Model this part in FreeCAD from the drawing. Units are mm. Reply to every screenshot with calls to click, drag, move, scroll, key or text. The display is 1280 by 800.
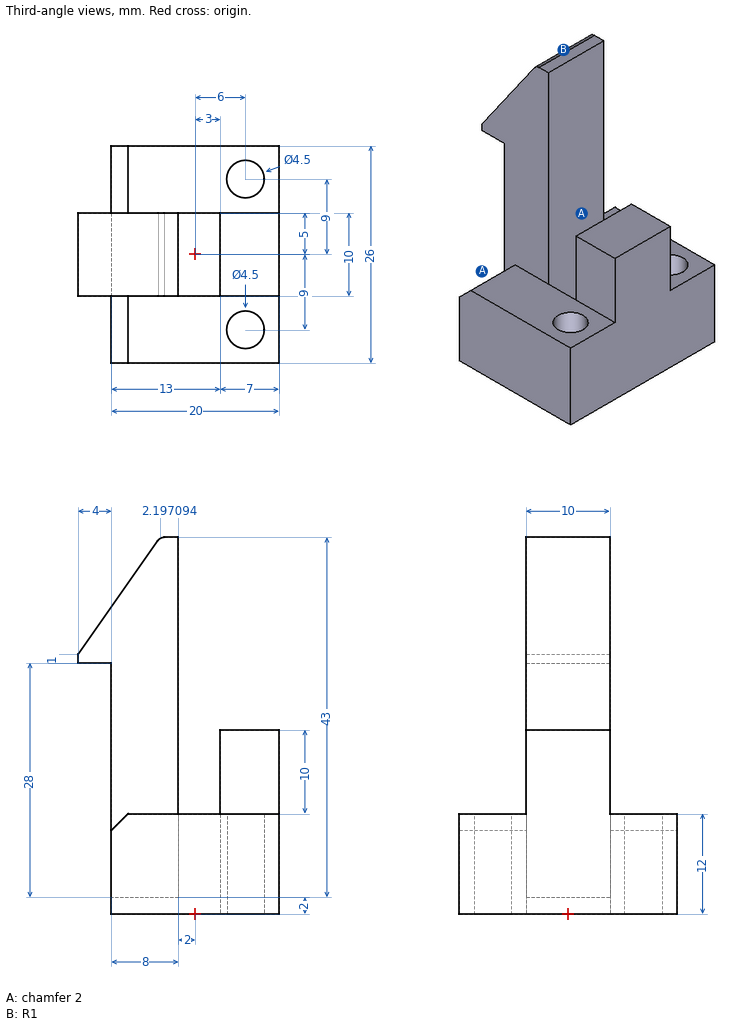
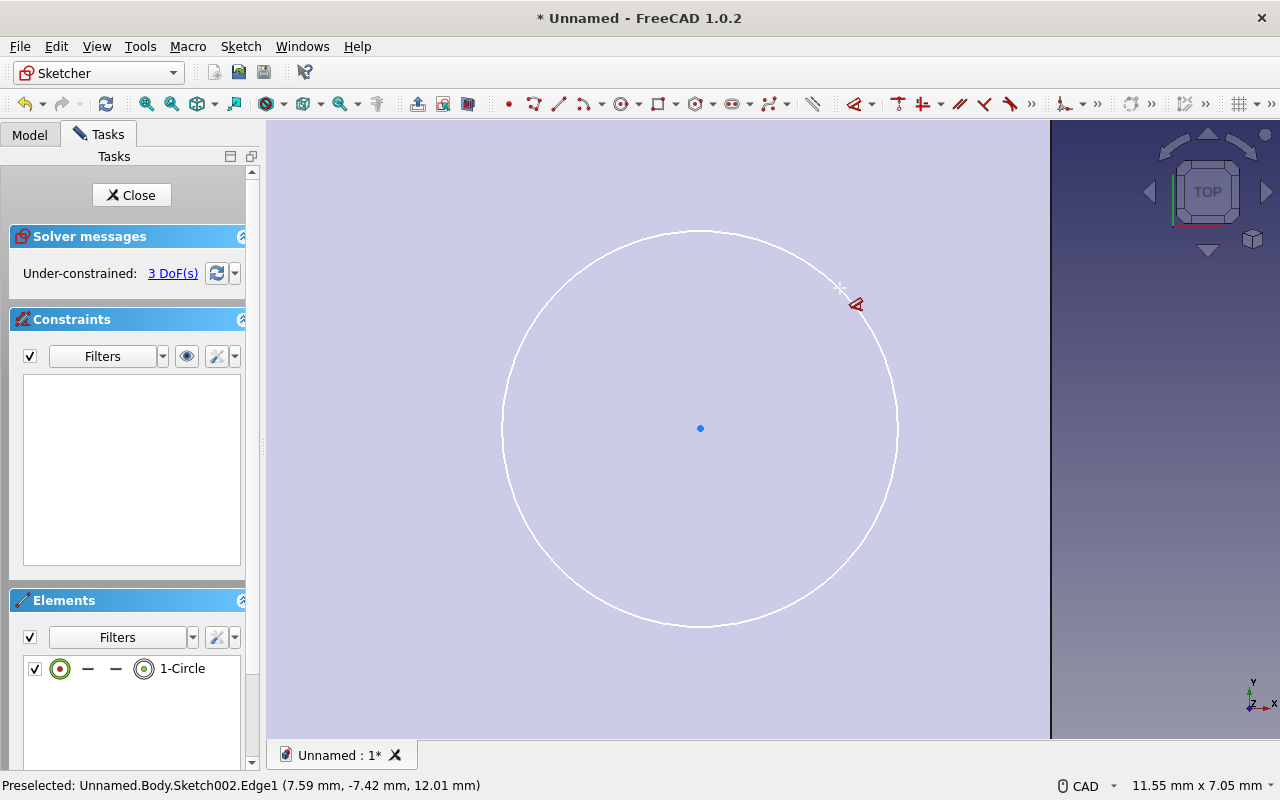
click(840, 289)
click(863, 266)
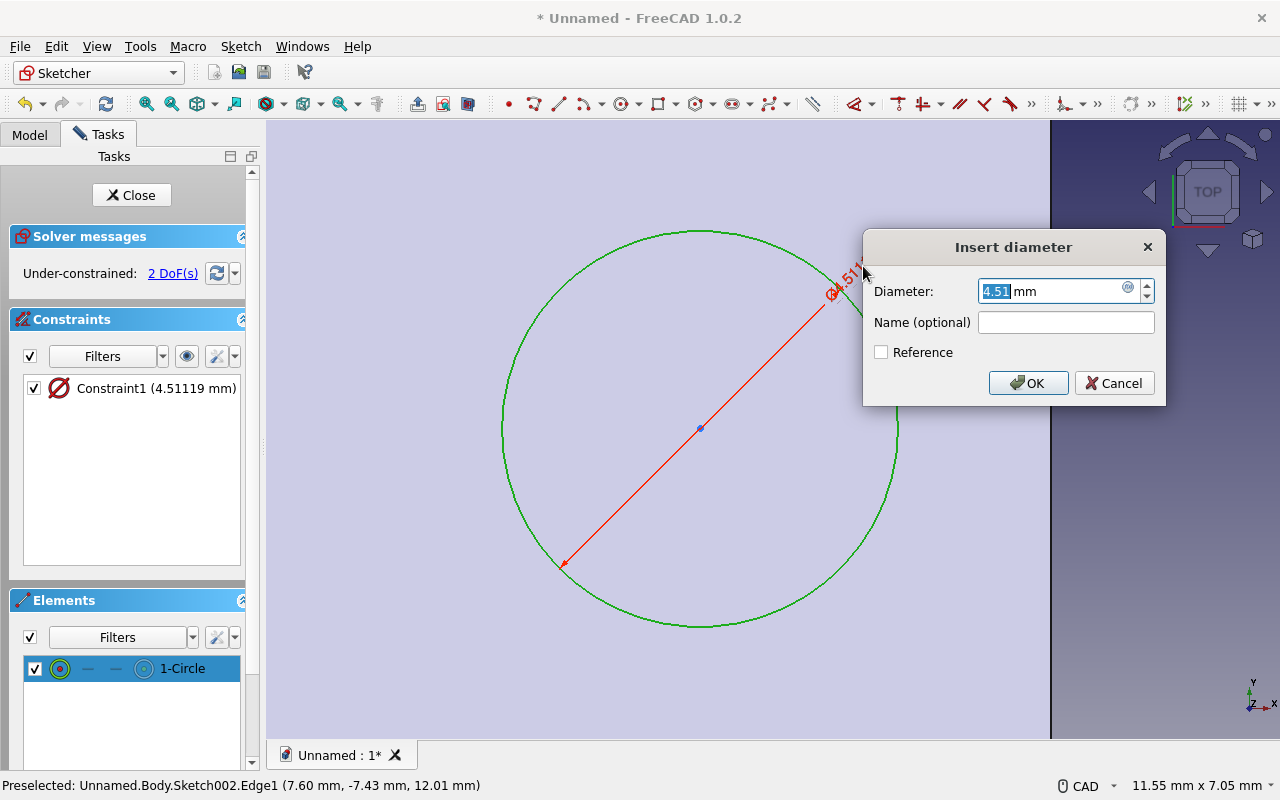
text(4.5)
key(Return)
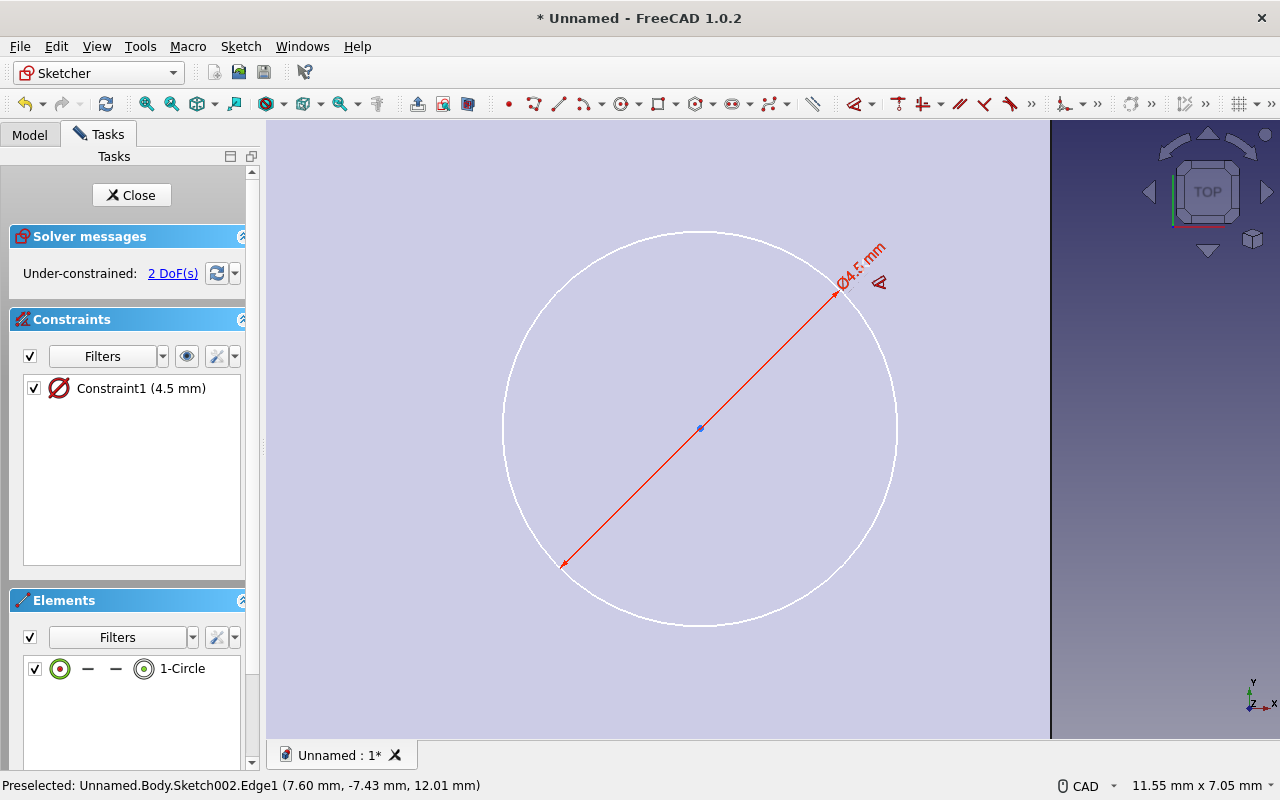
click(700, 429)
click(404, 463)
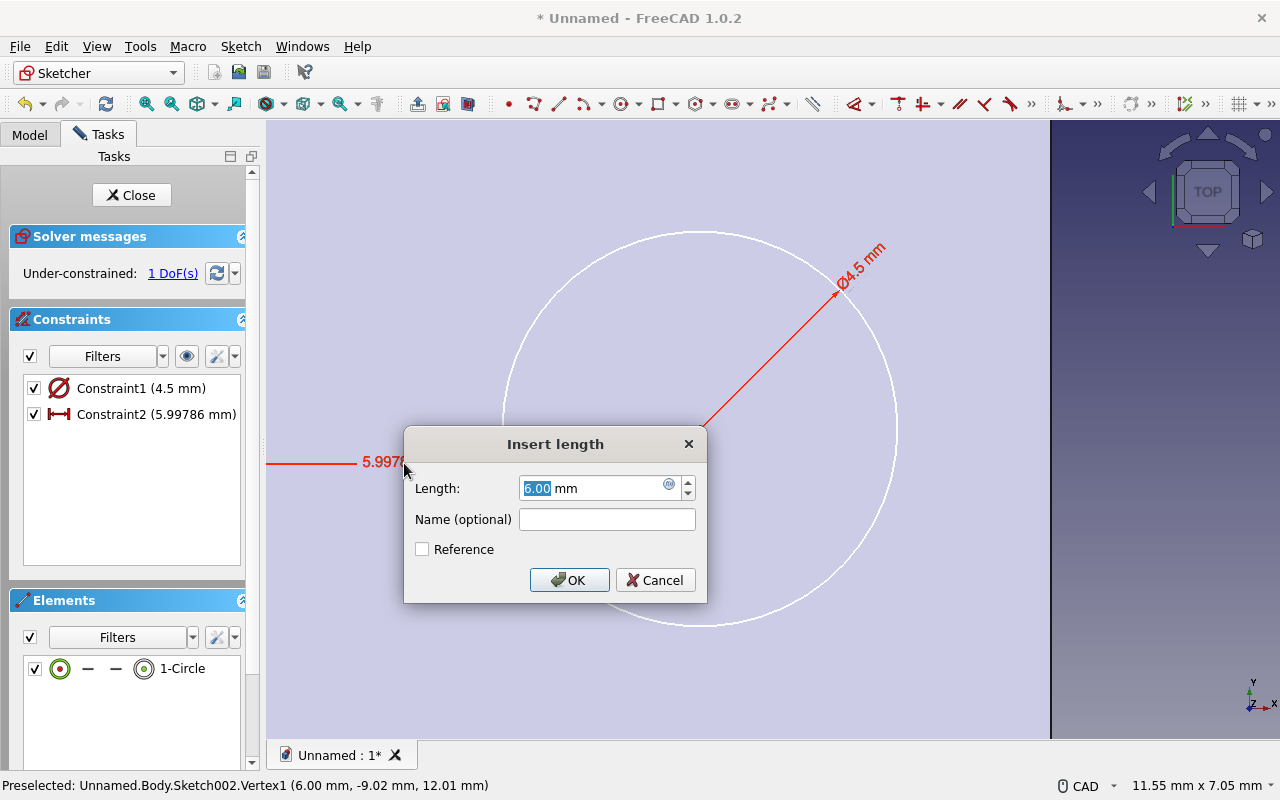
text(6)
key(Return)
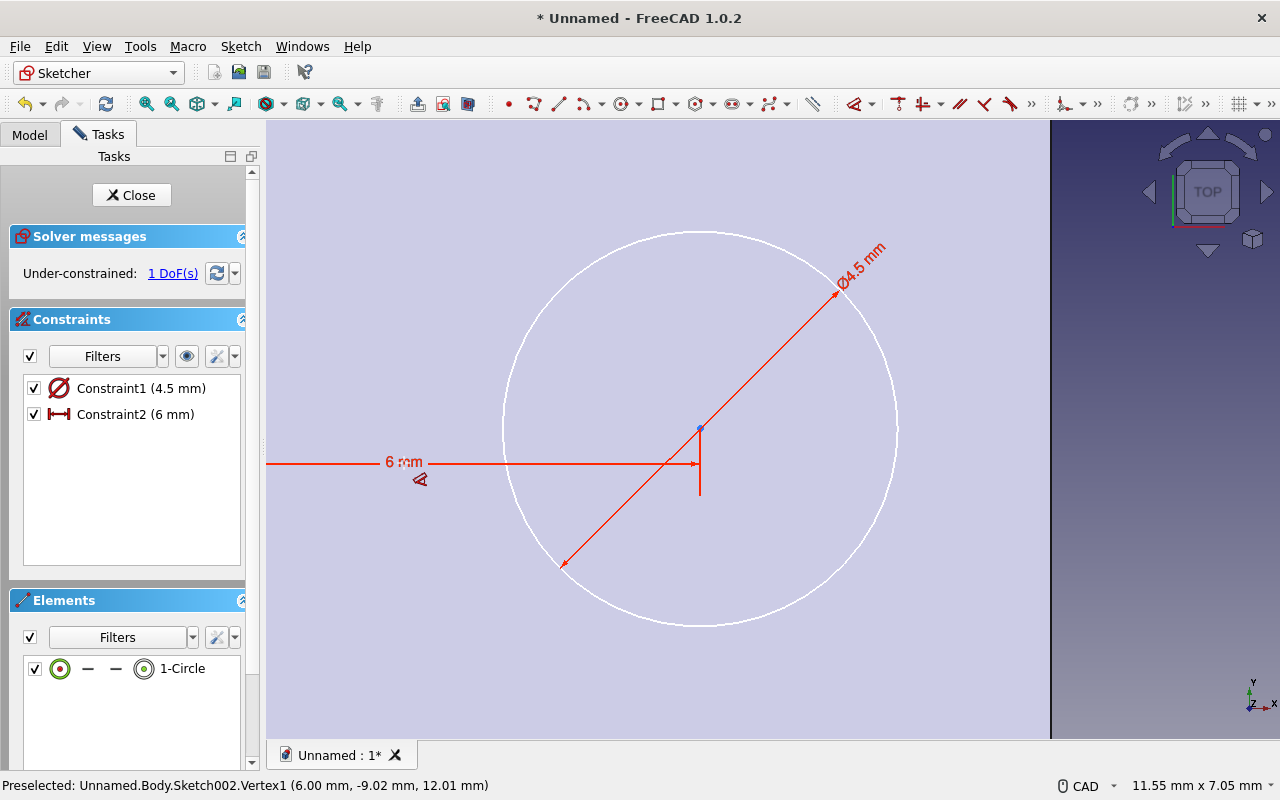
click(700, 429)
click(734, 288)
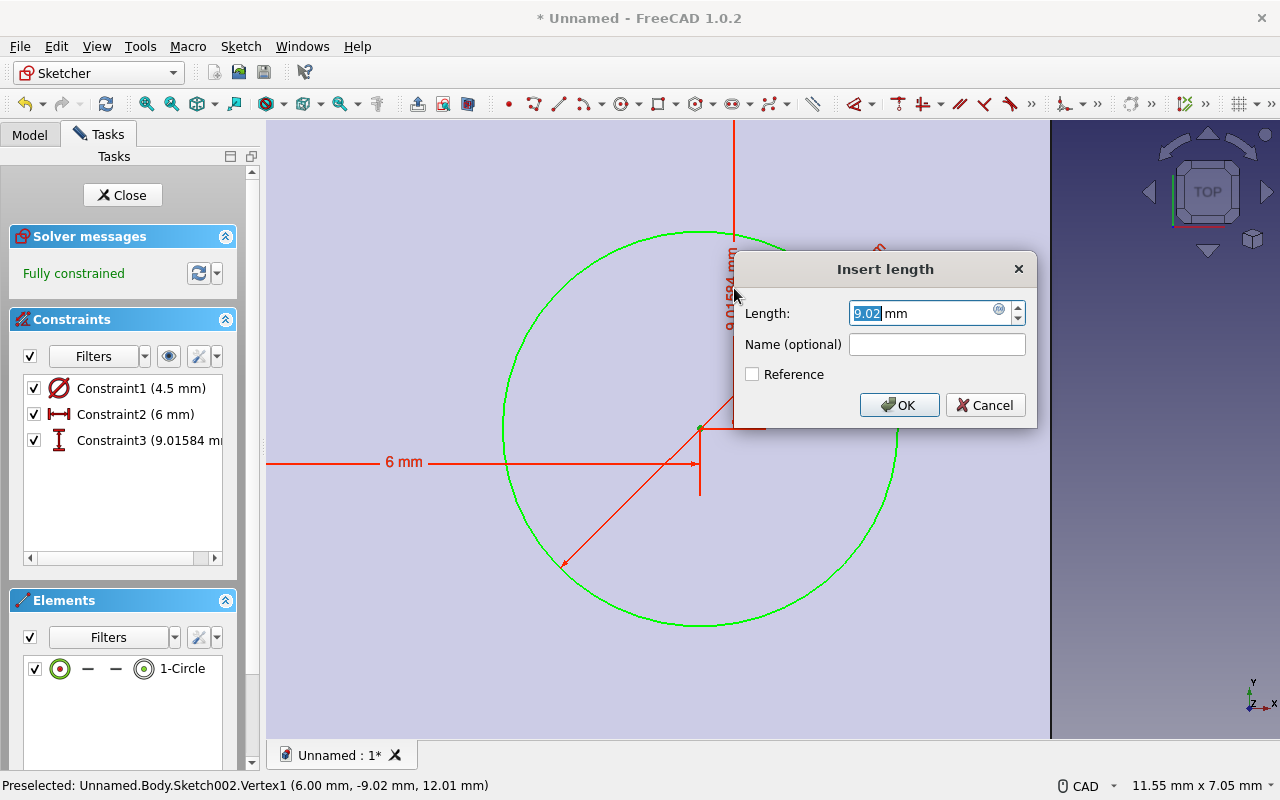
text(9)
key(Return)
key(Escape)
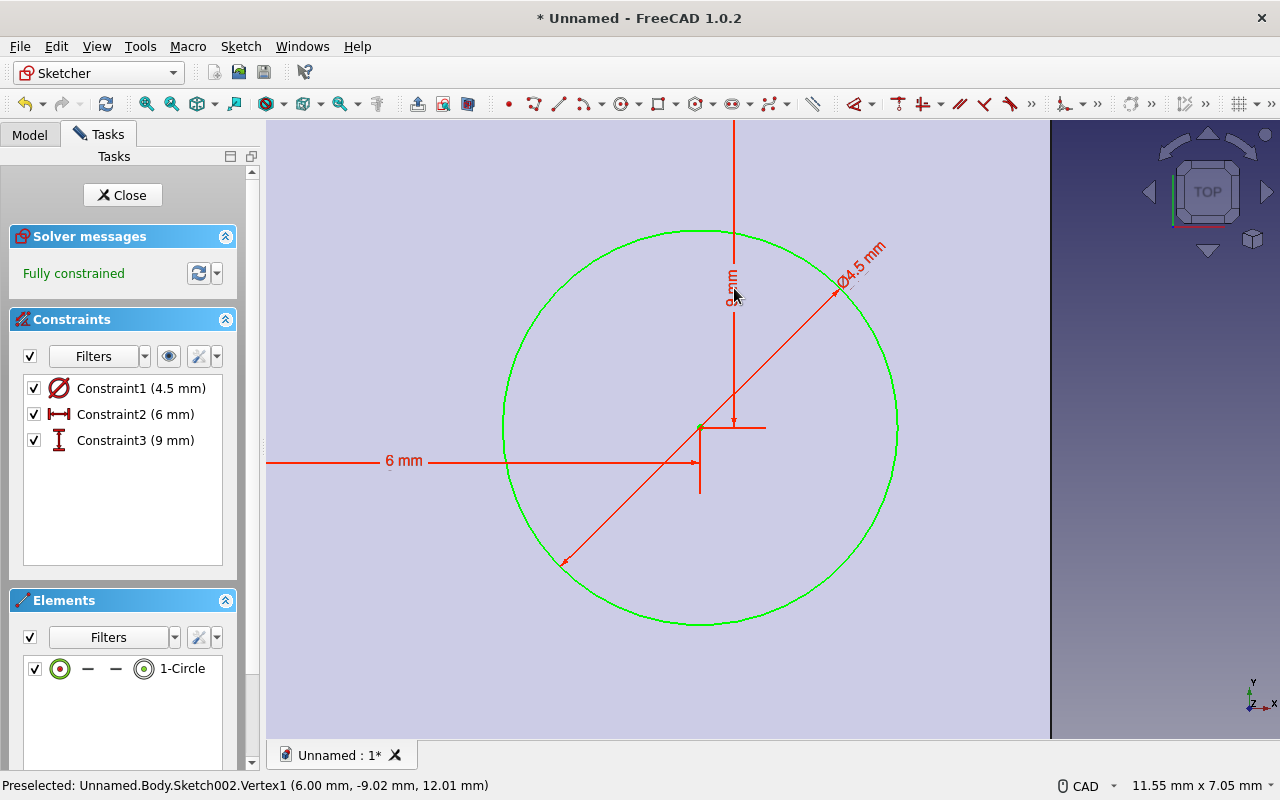
click(123, 195)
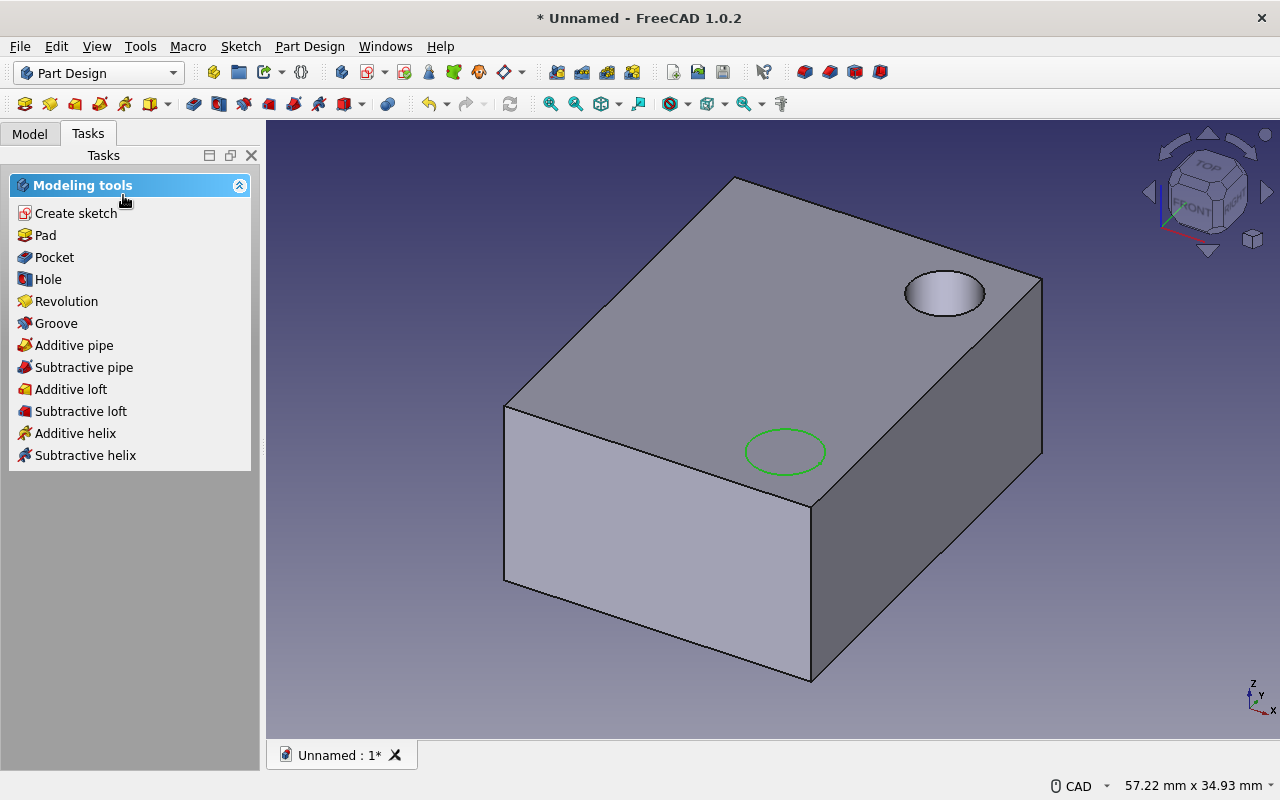
click(194, 104)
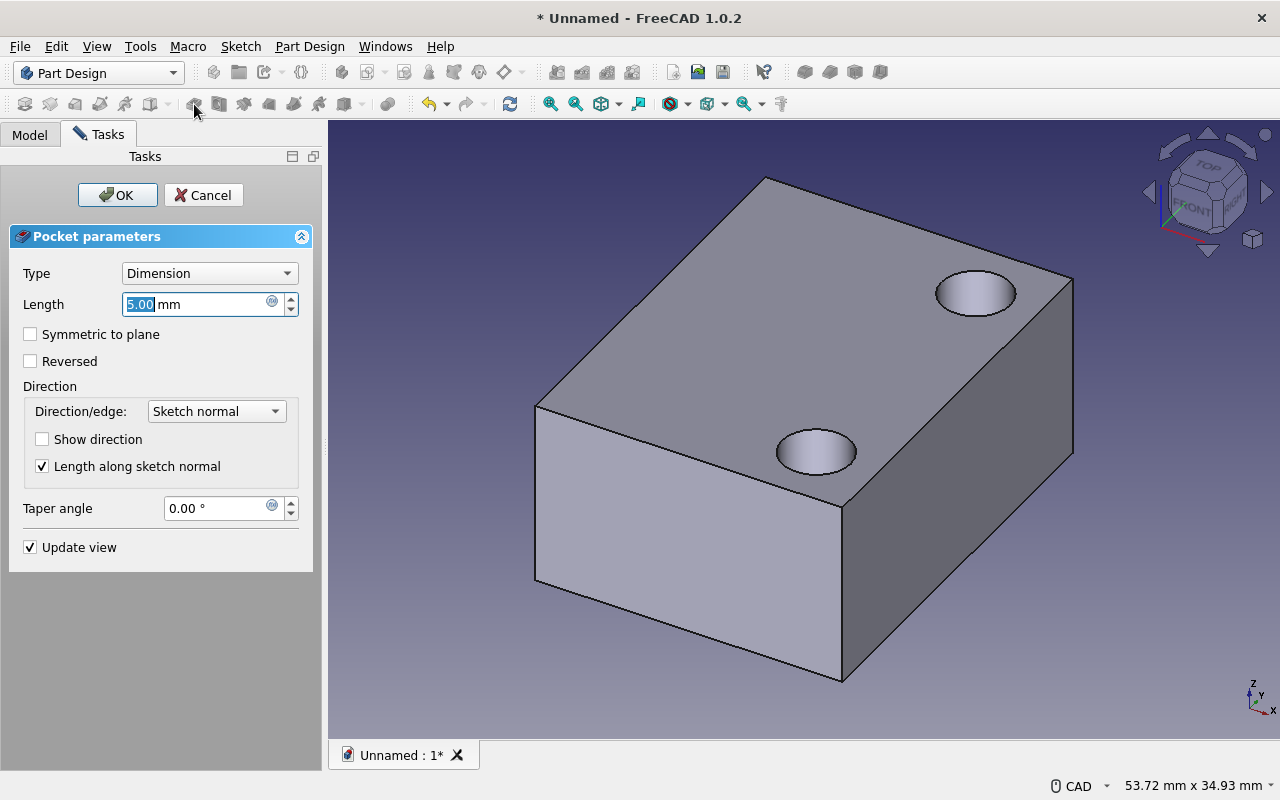
click(210, 274)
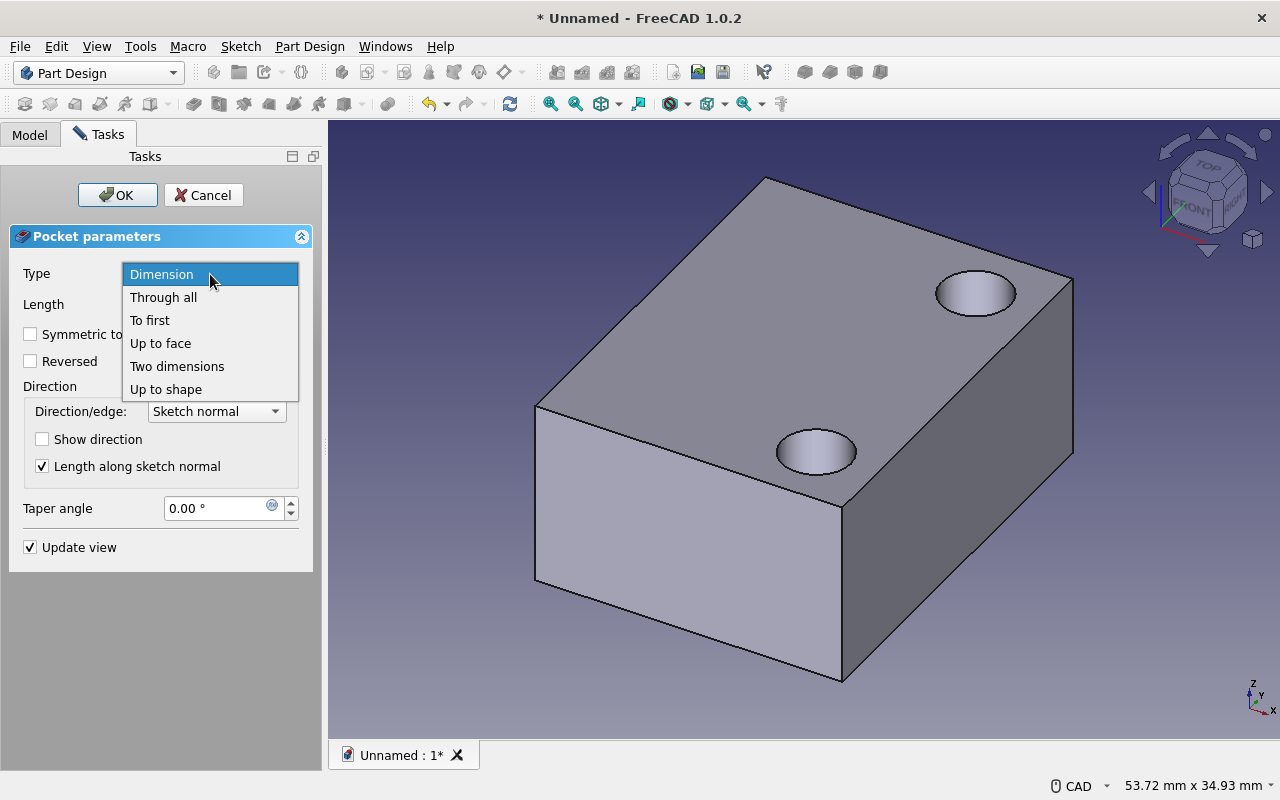
click(208, 320)